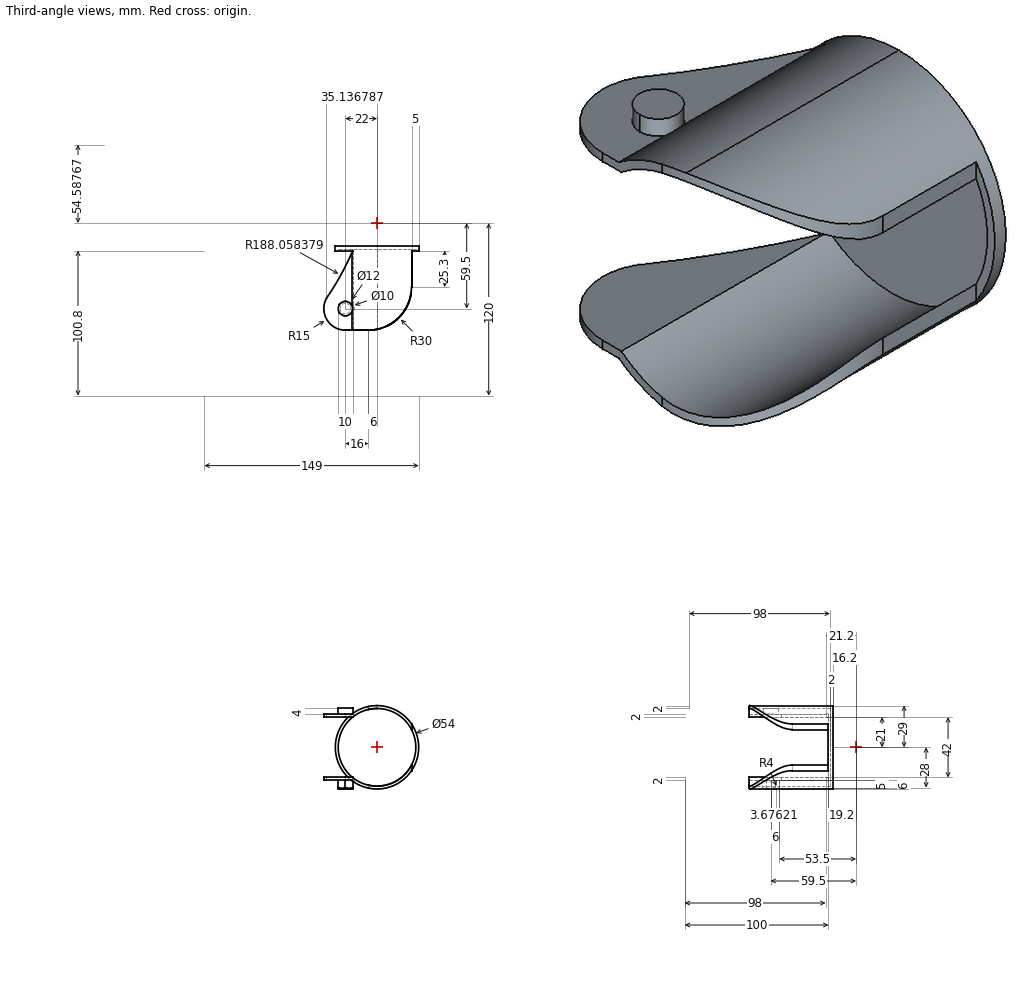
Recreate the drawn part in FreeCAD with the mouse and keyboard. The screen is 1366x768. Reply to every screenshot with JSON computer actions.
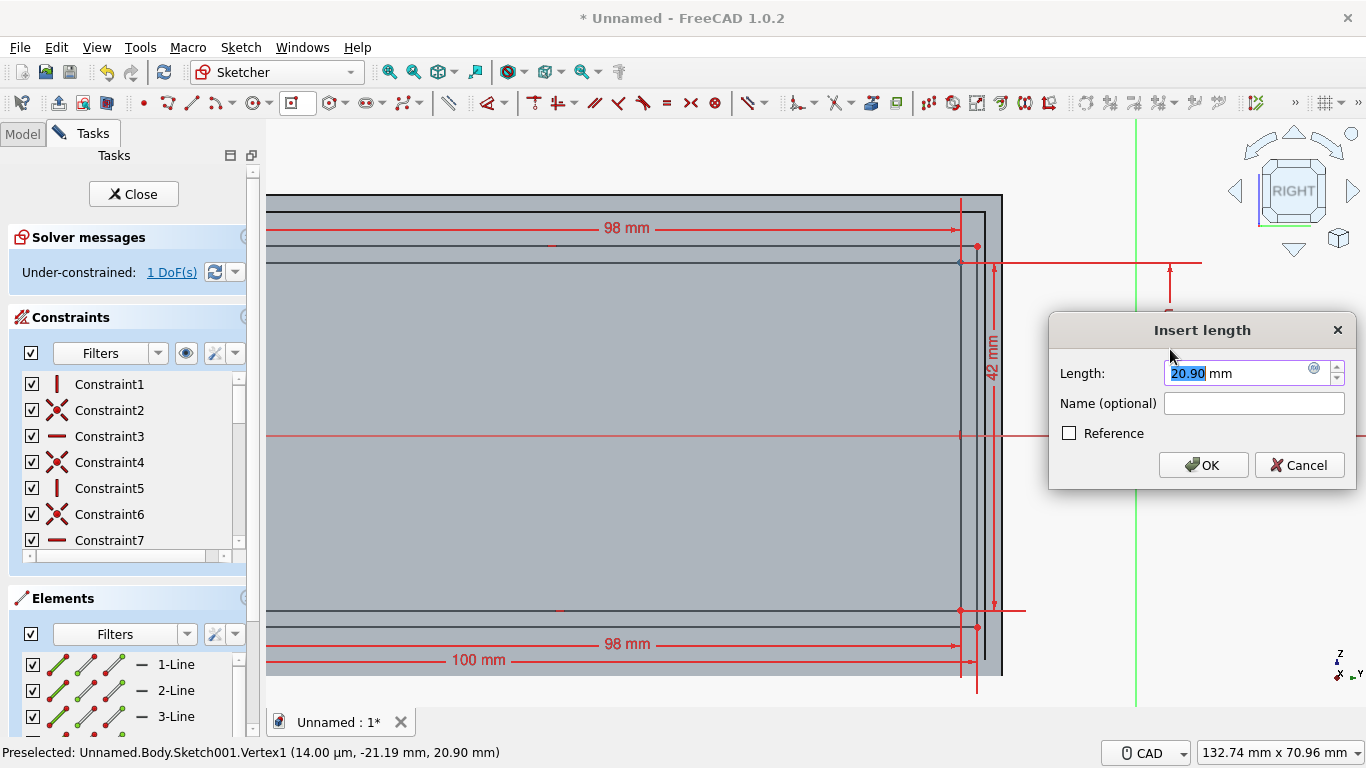
{"action": "type", "text": "21"}
{"action": "key", "text": "Return"}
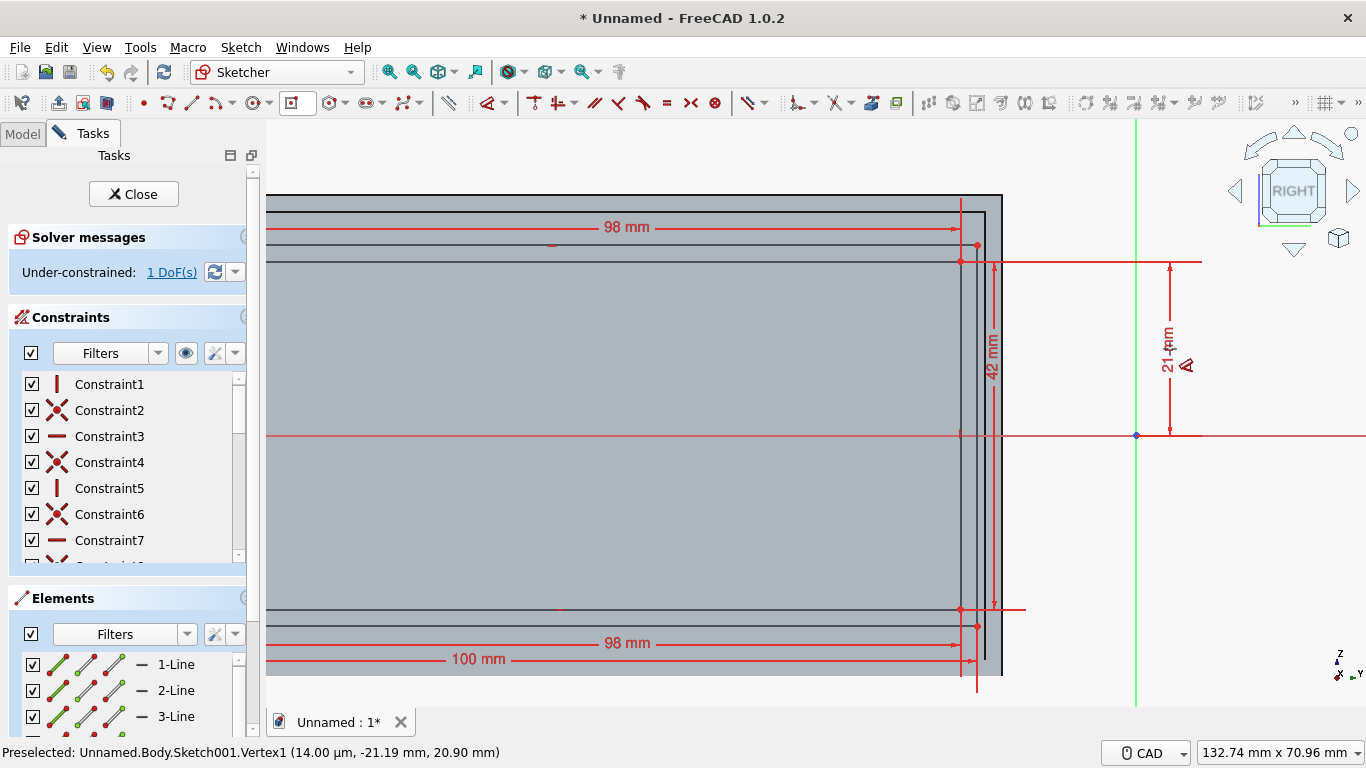
{"action": "left_click", "coordinate": [961, 262]}
{"action": "left_click", "coordinate": [1048, 228]}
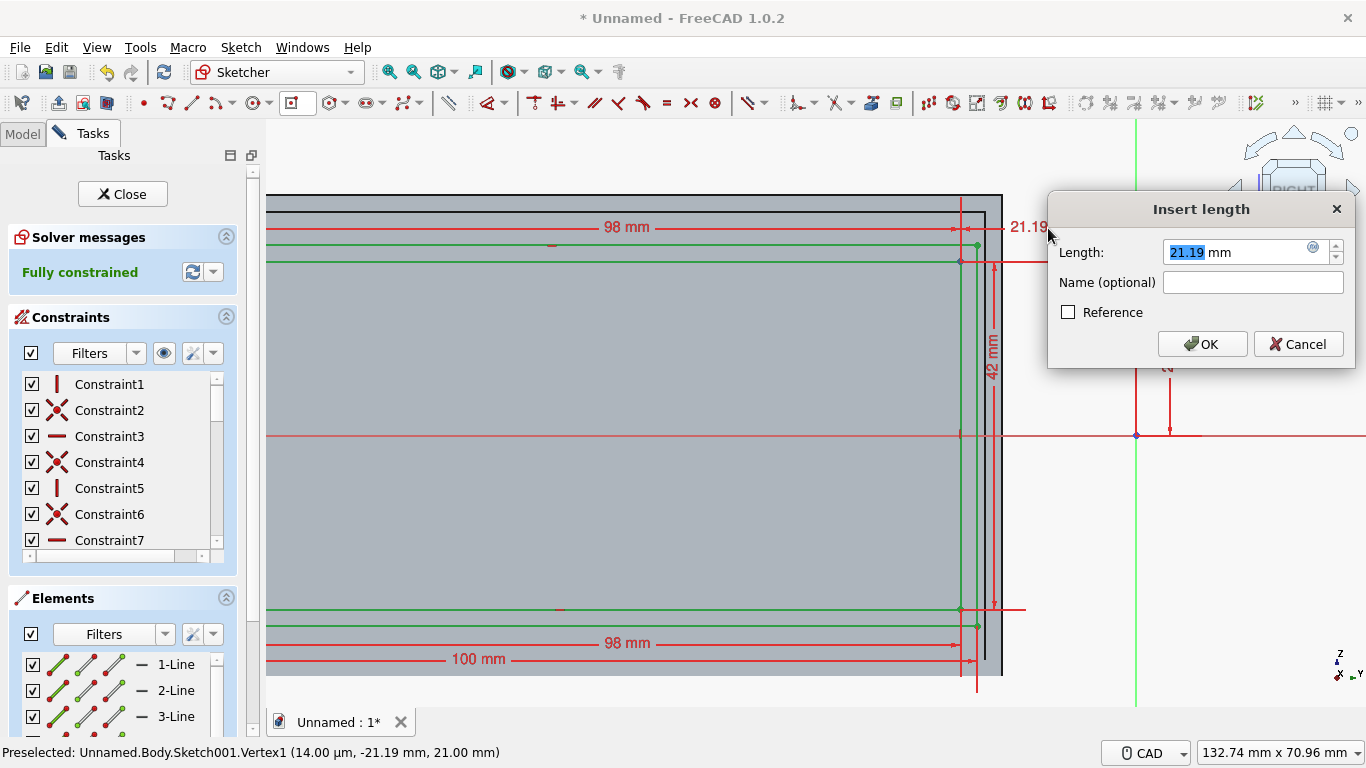
{"action": "type", "text": "21.2"}
{"action": "key", "text": "Return"}
{"action": "key", "text": "Escape"}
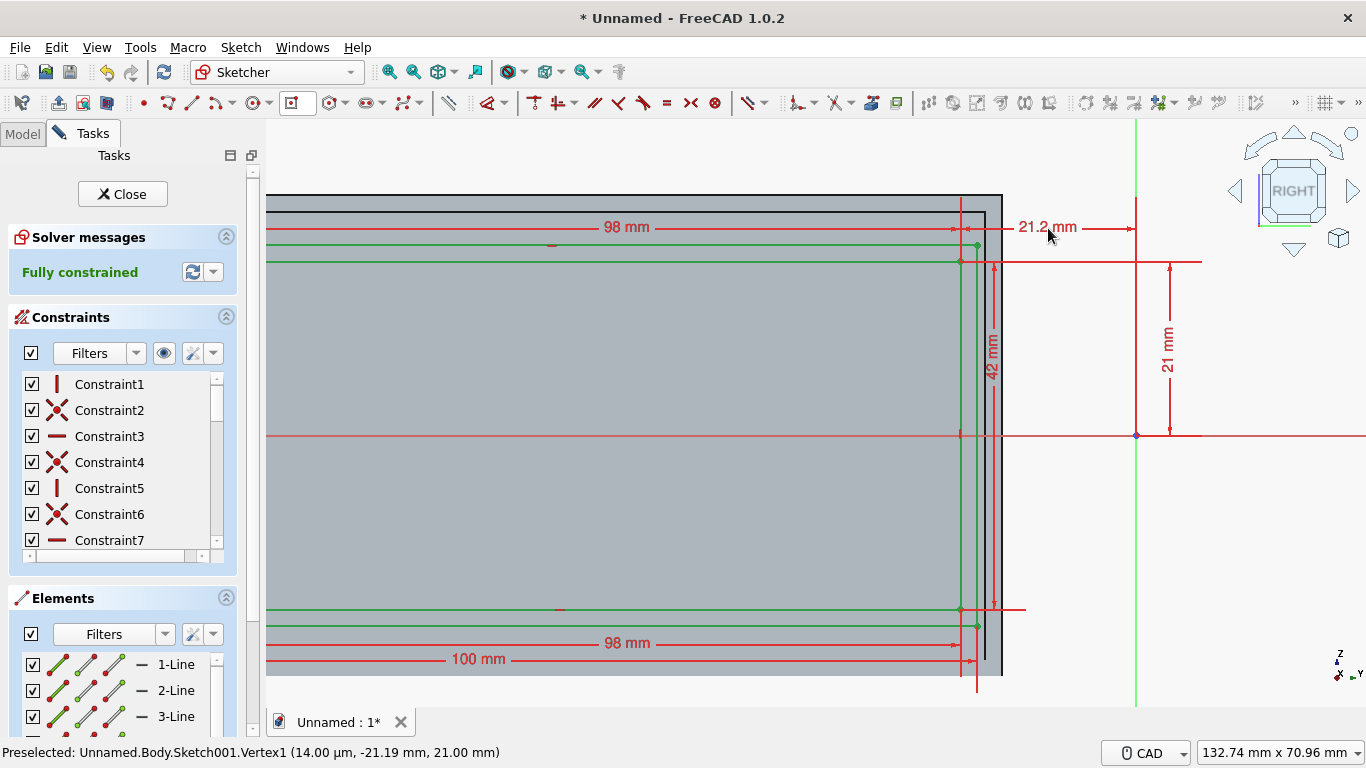
{"action": "left_click", "coordinate": [123, 194]}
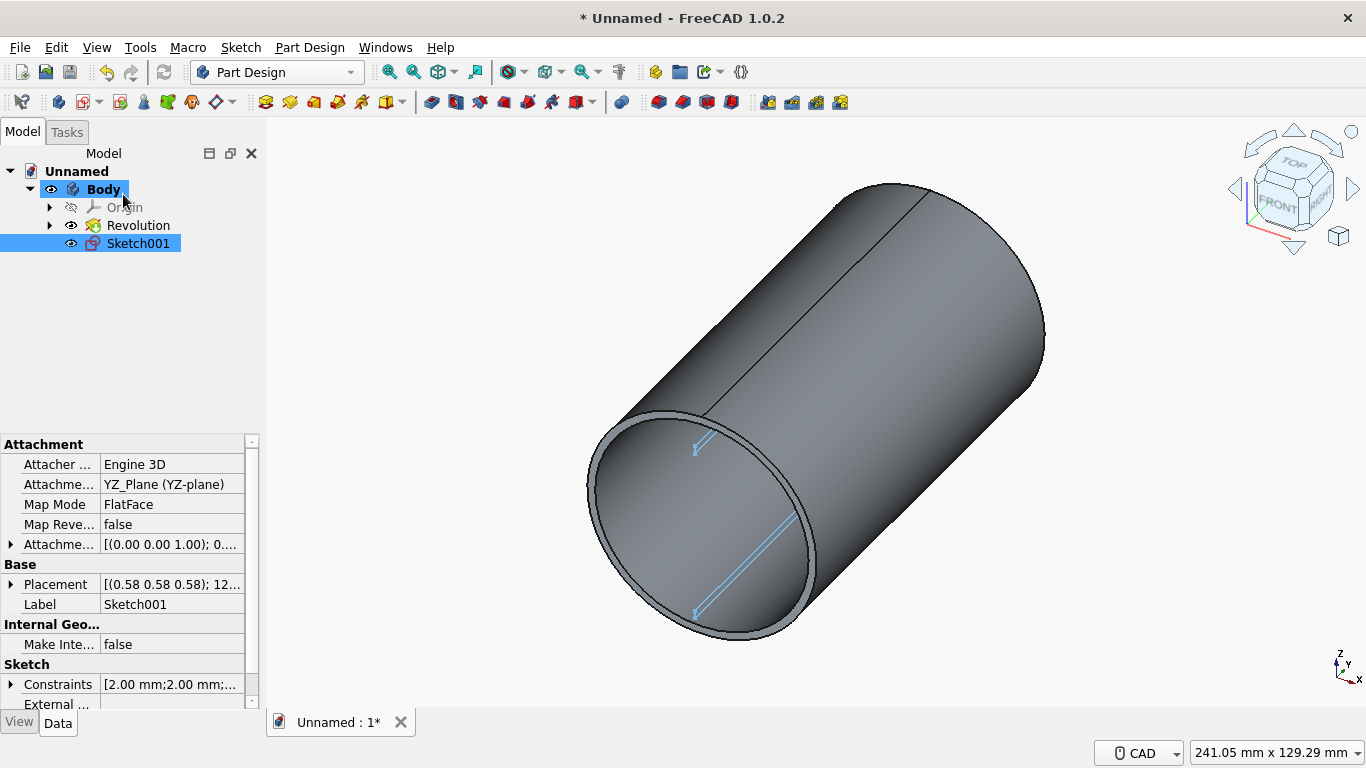
{"action": "left_click", "coordinate": [266, 102]}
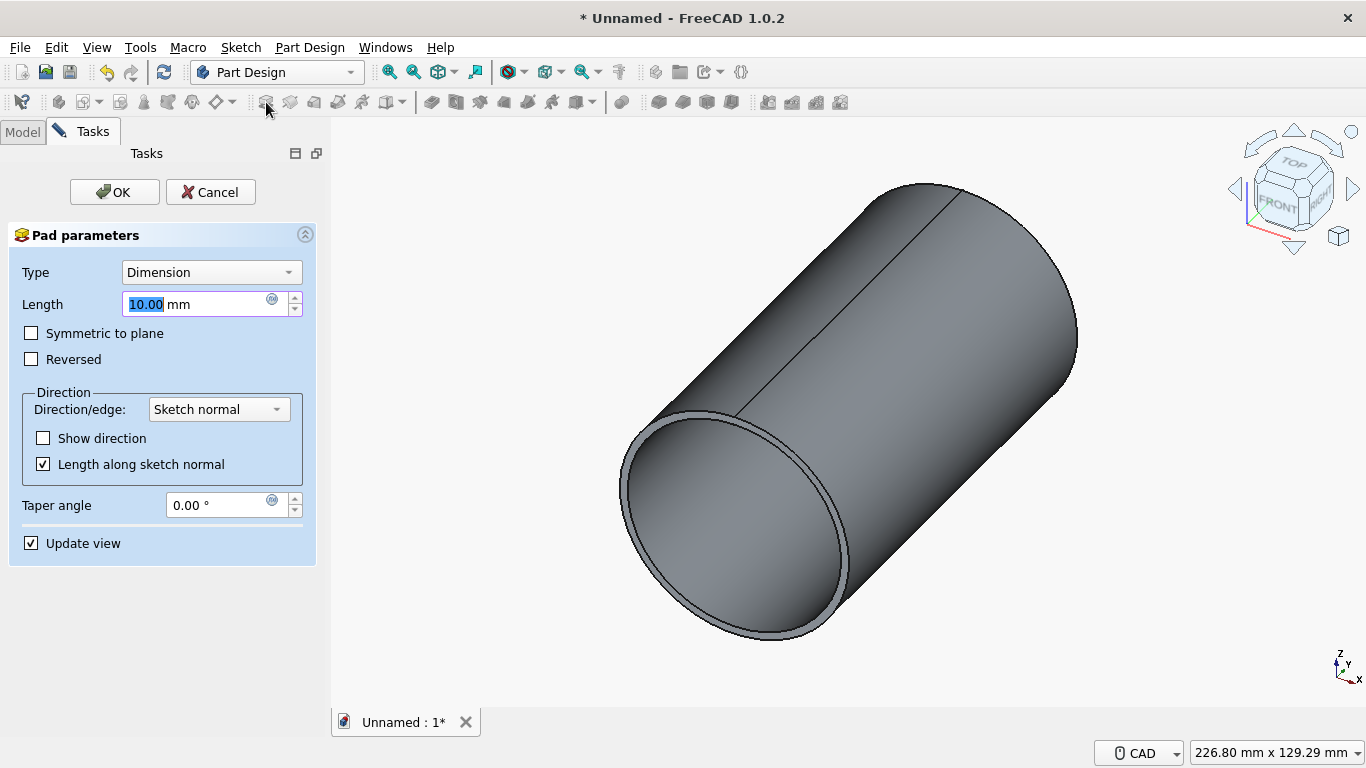
{"action": "type", "text": "100"}
{"action": "key", "text": "Tab"}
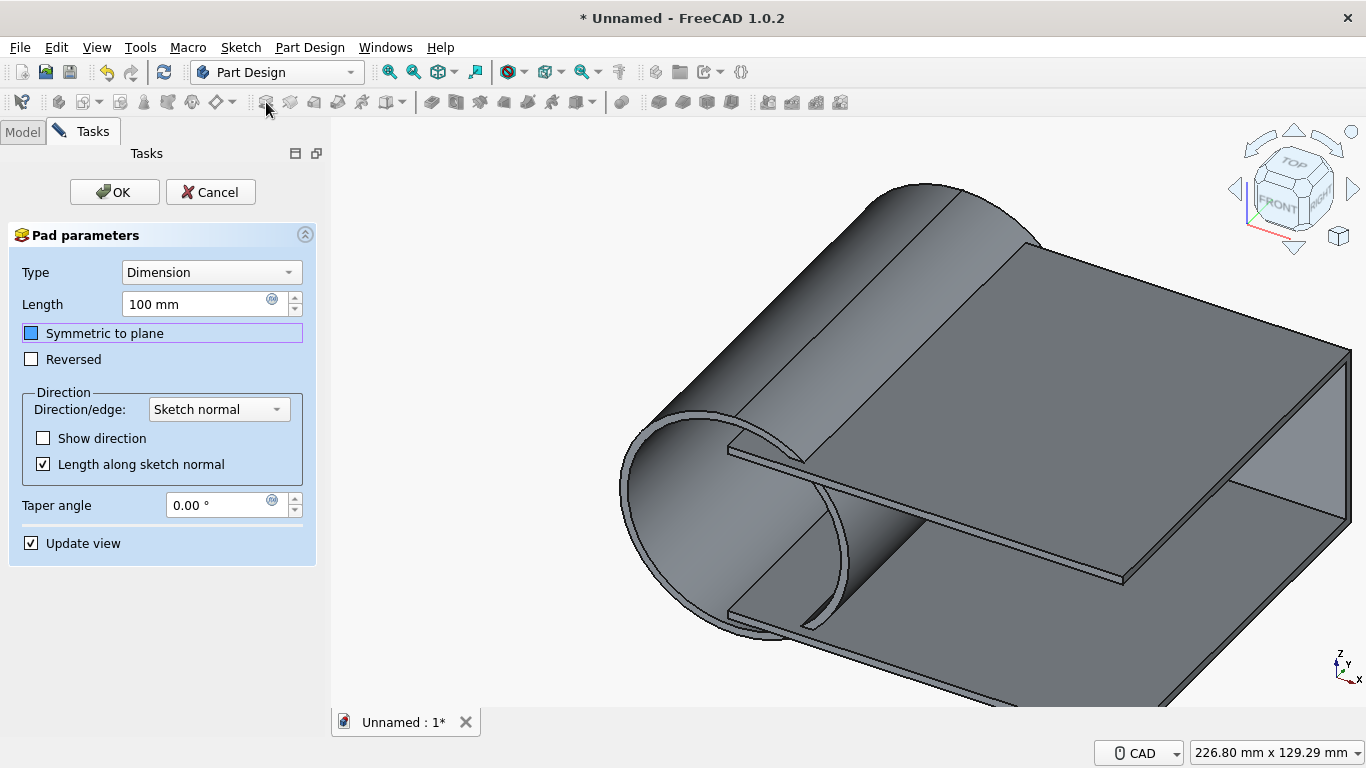
{"action": "left_click", "coordinate": [30, 359]}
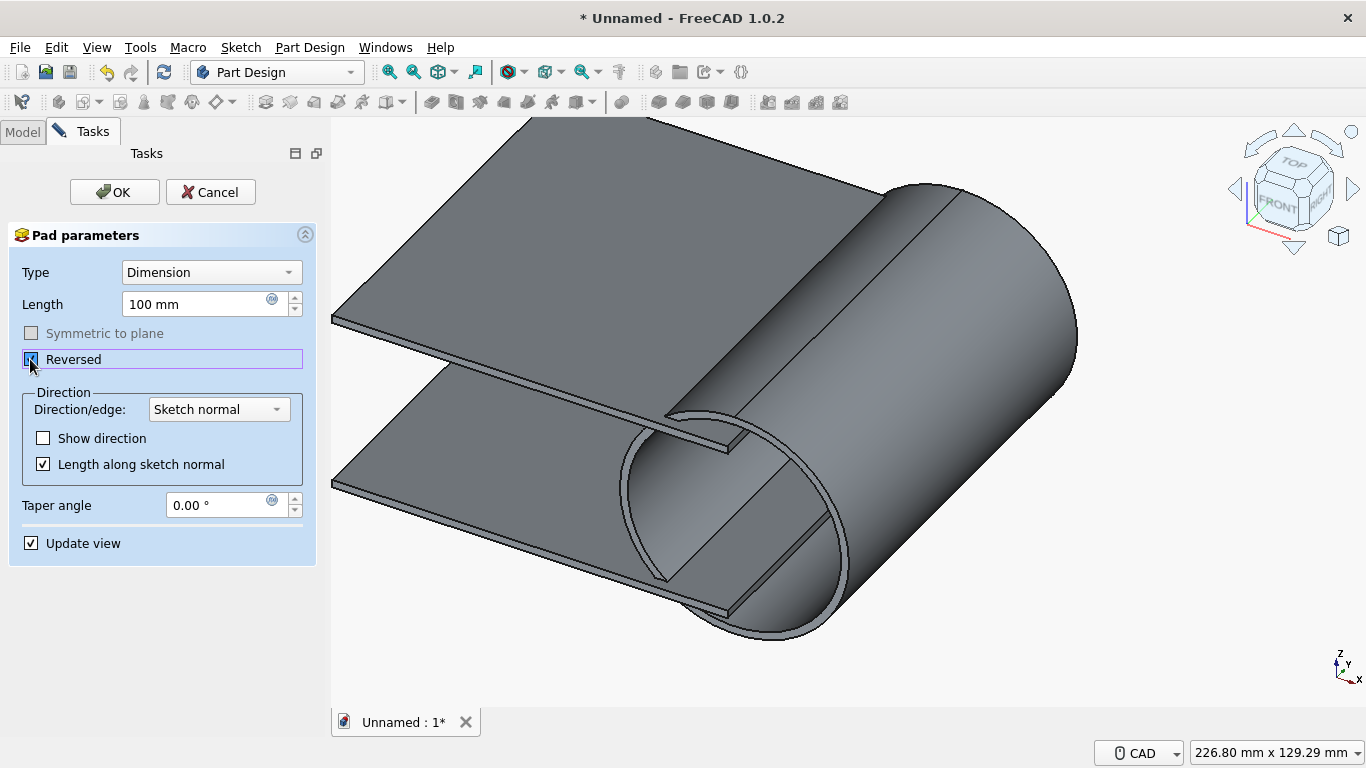
{"action": "left_click", "coordinate": [115, 192]}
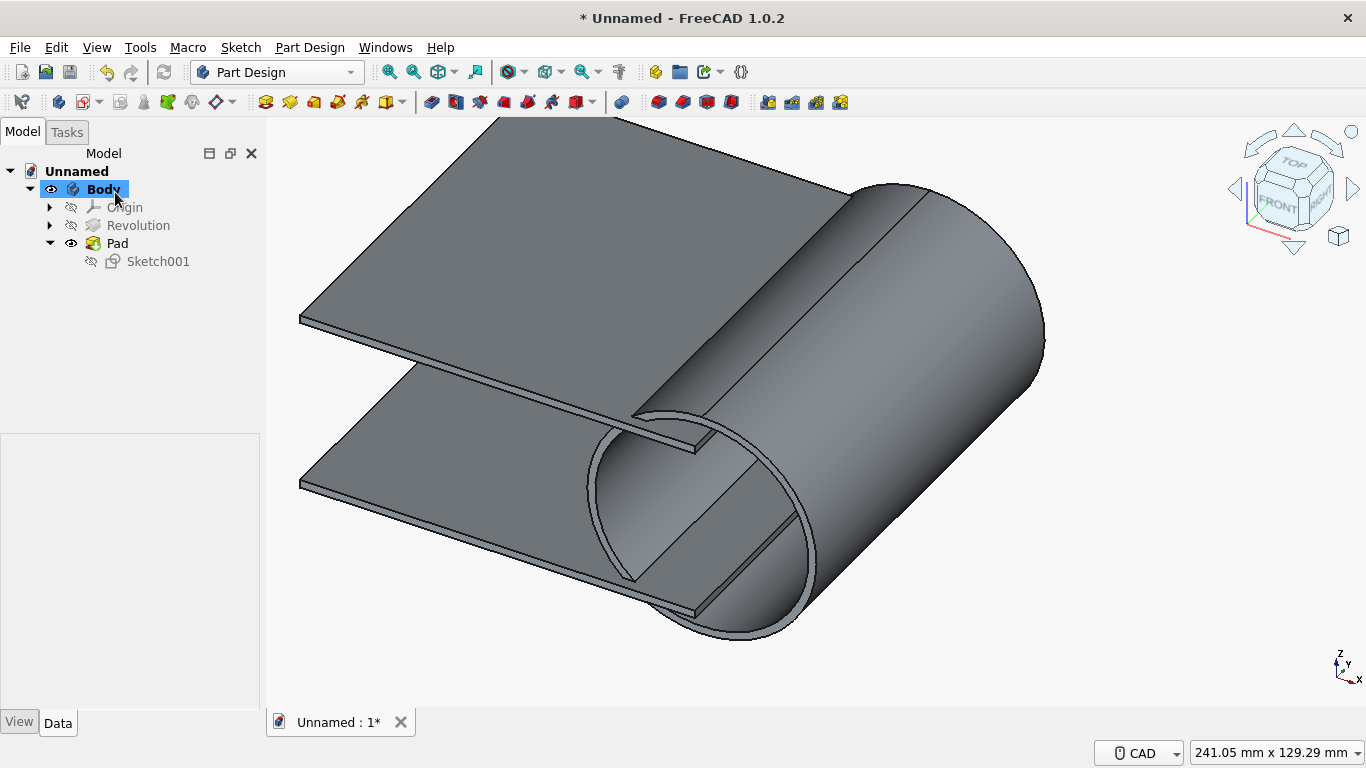
{"action": "left_click", "coordinate": [390, 72]}